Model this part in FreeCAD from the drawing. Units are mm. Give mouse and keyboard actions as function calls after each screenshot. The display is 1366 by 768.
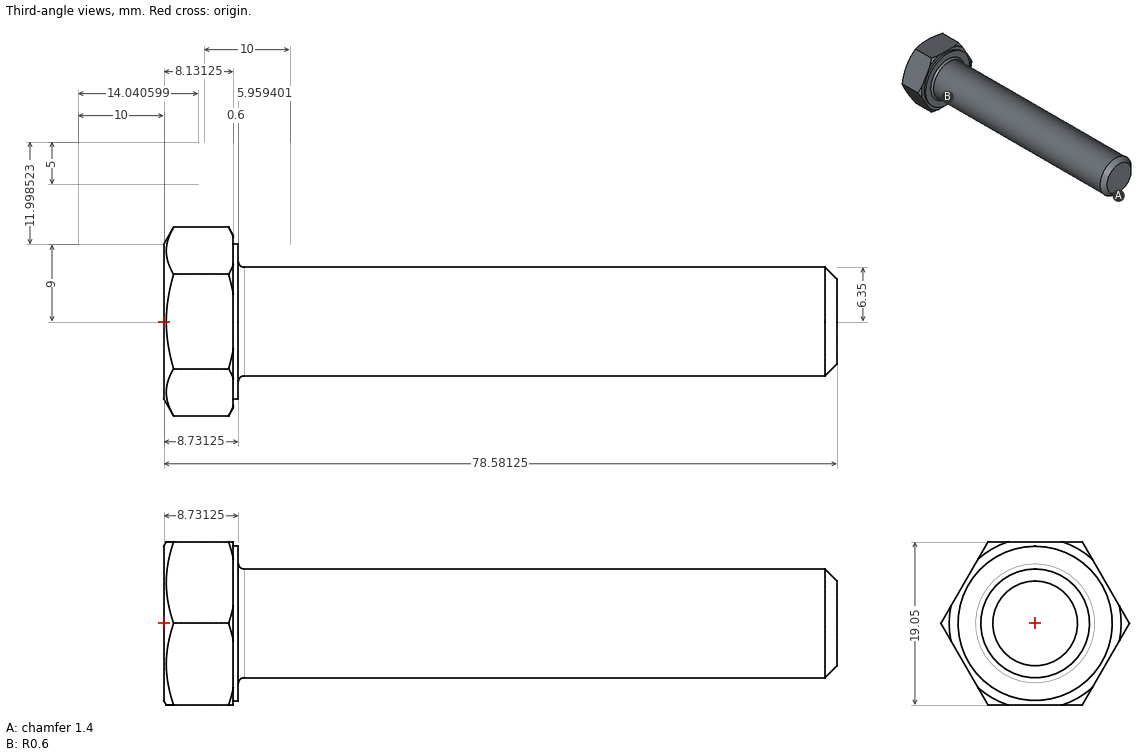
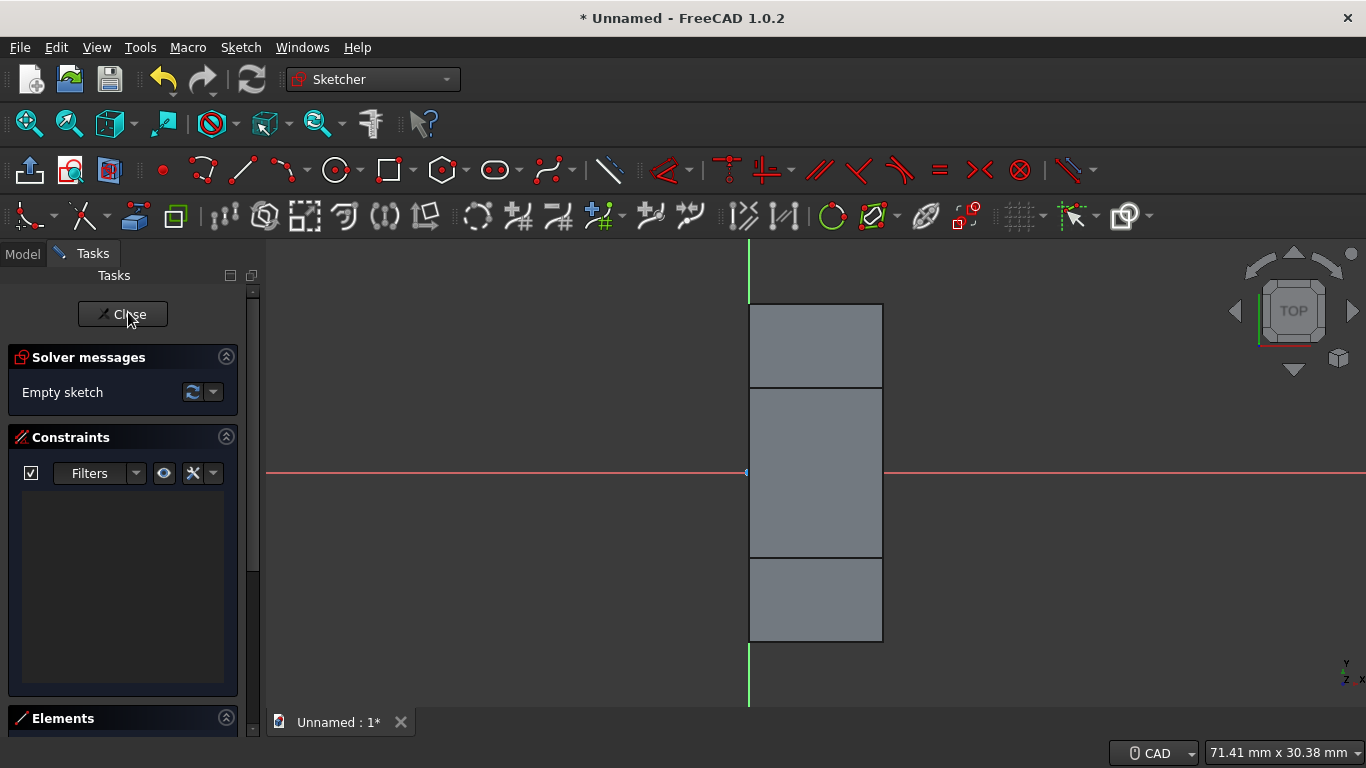
click(110, 170)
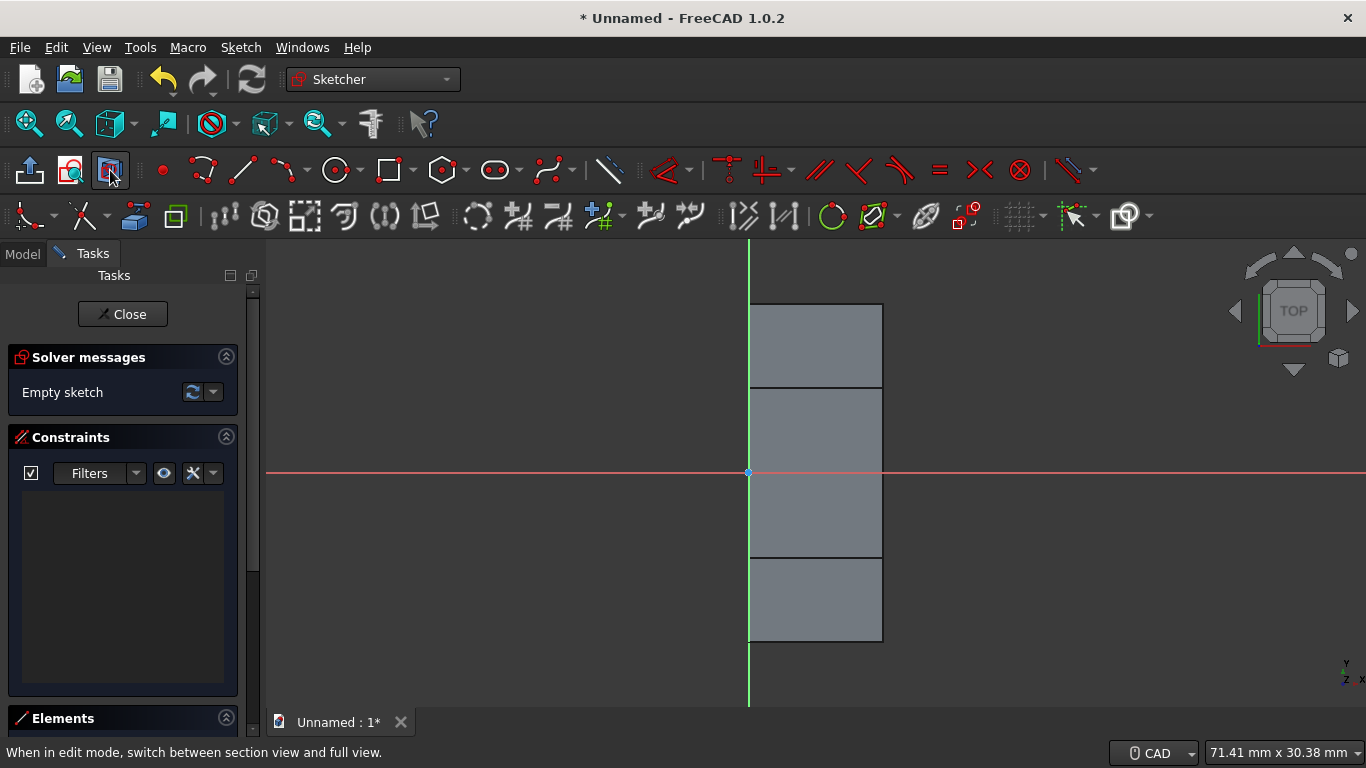
scroll(294, 513, down, 4)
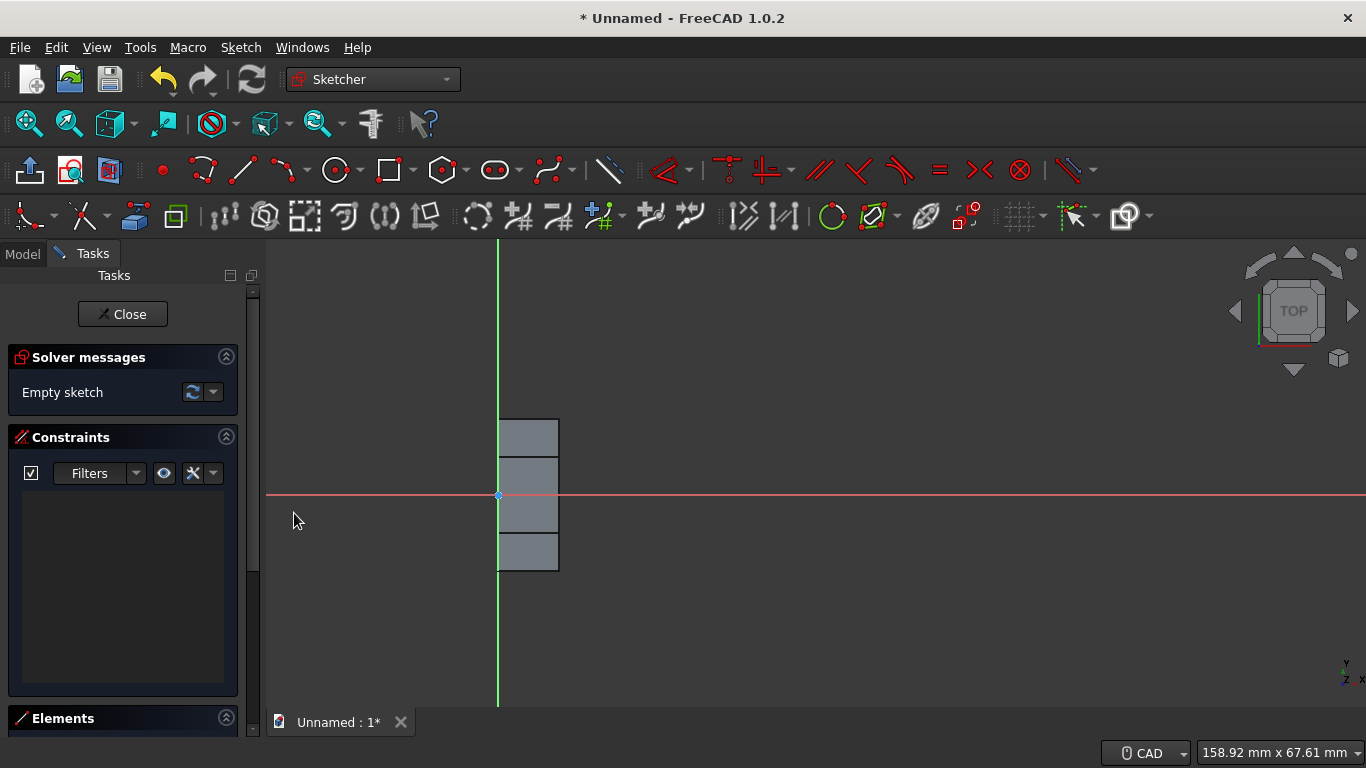
click(390, 170)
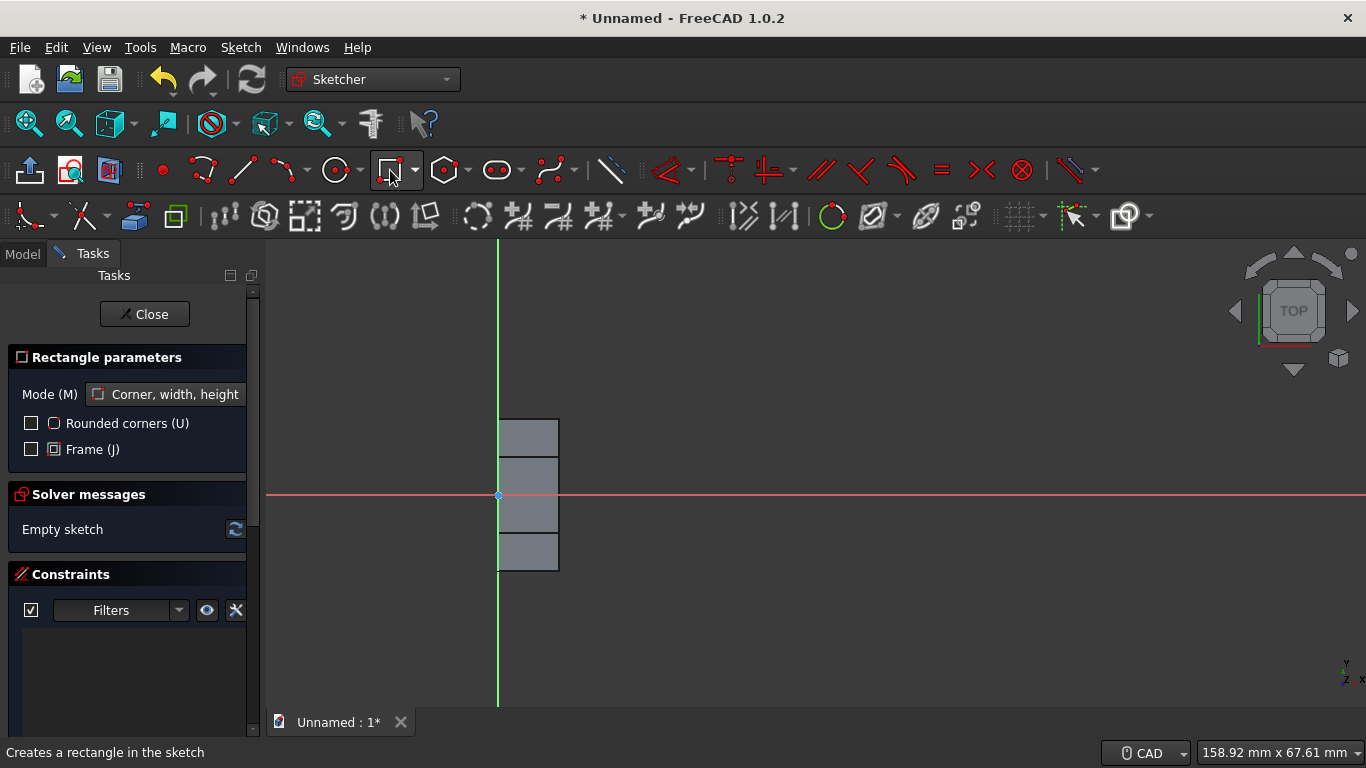
click(498, 495)
move(1042, 451)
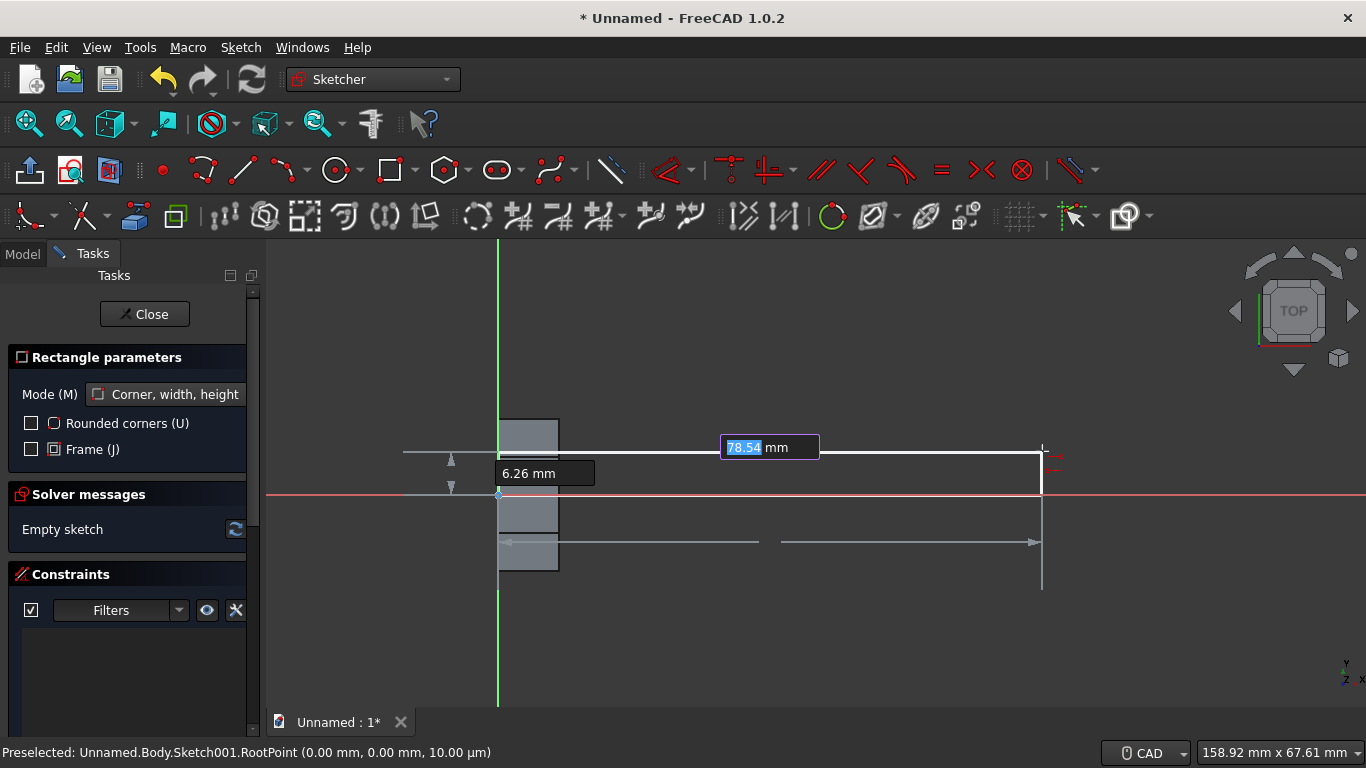
text(78.58125)
key(Tab)
text(6.35)
key(Return)
key(Escape)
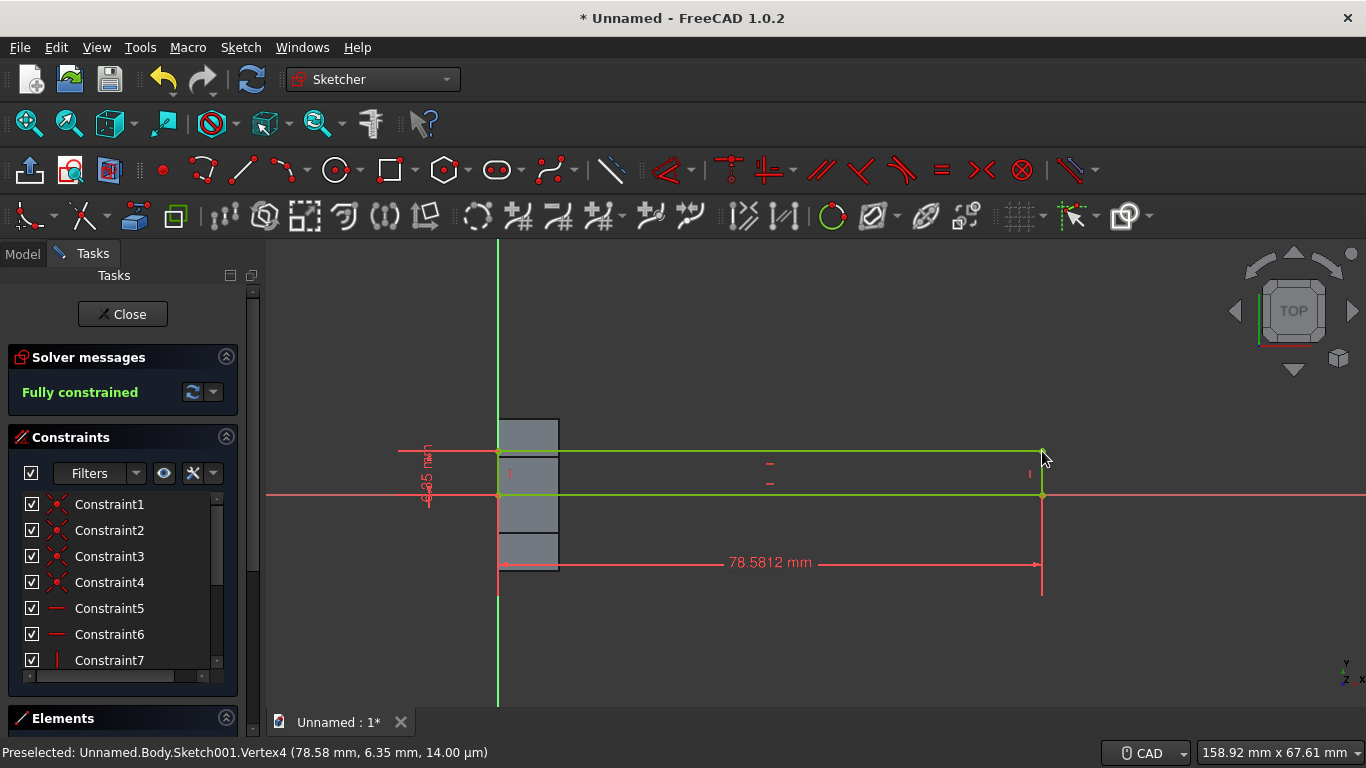
click(123, 314)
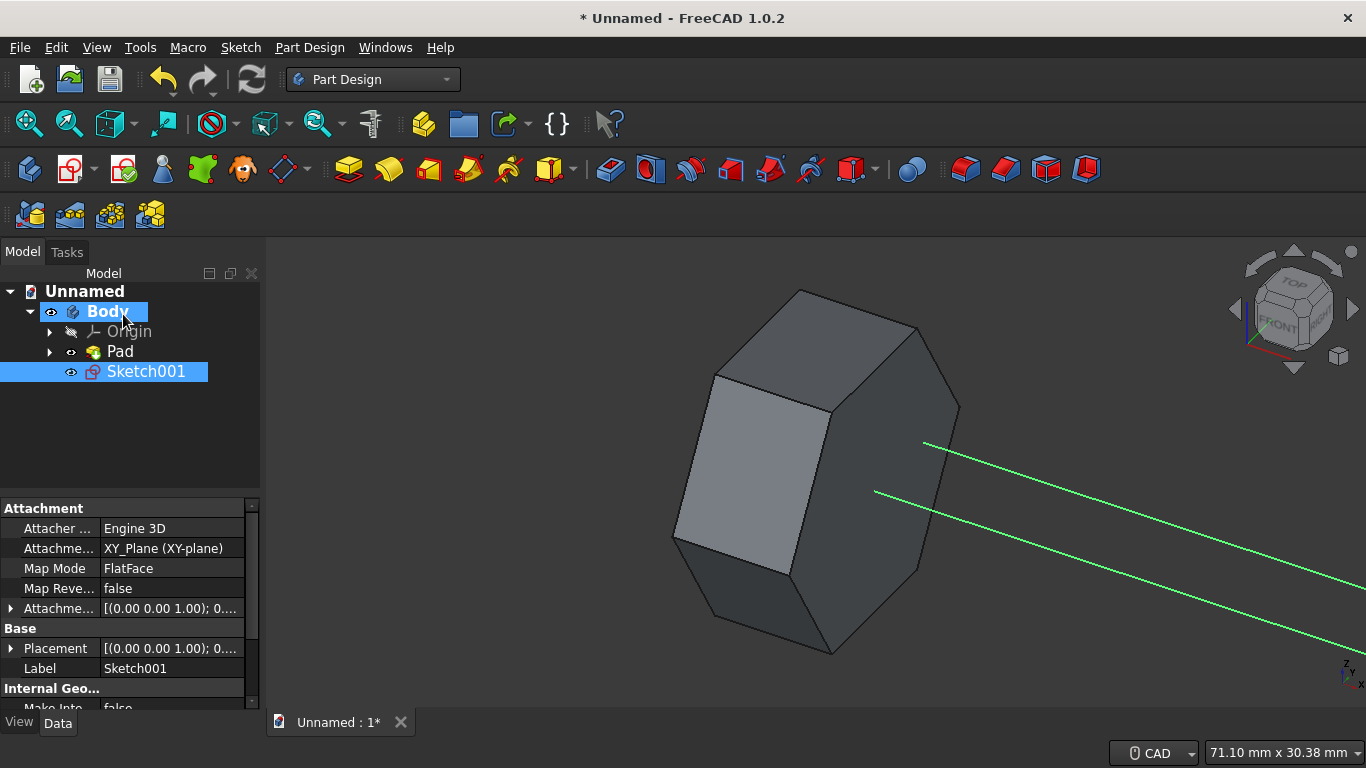
click(390, 170)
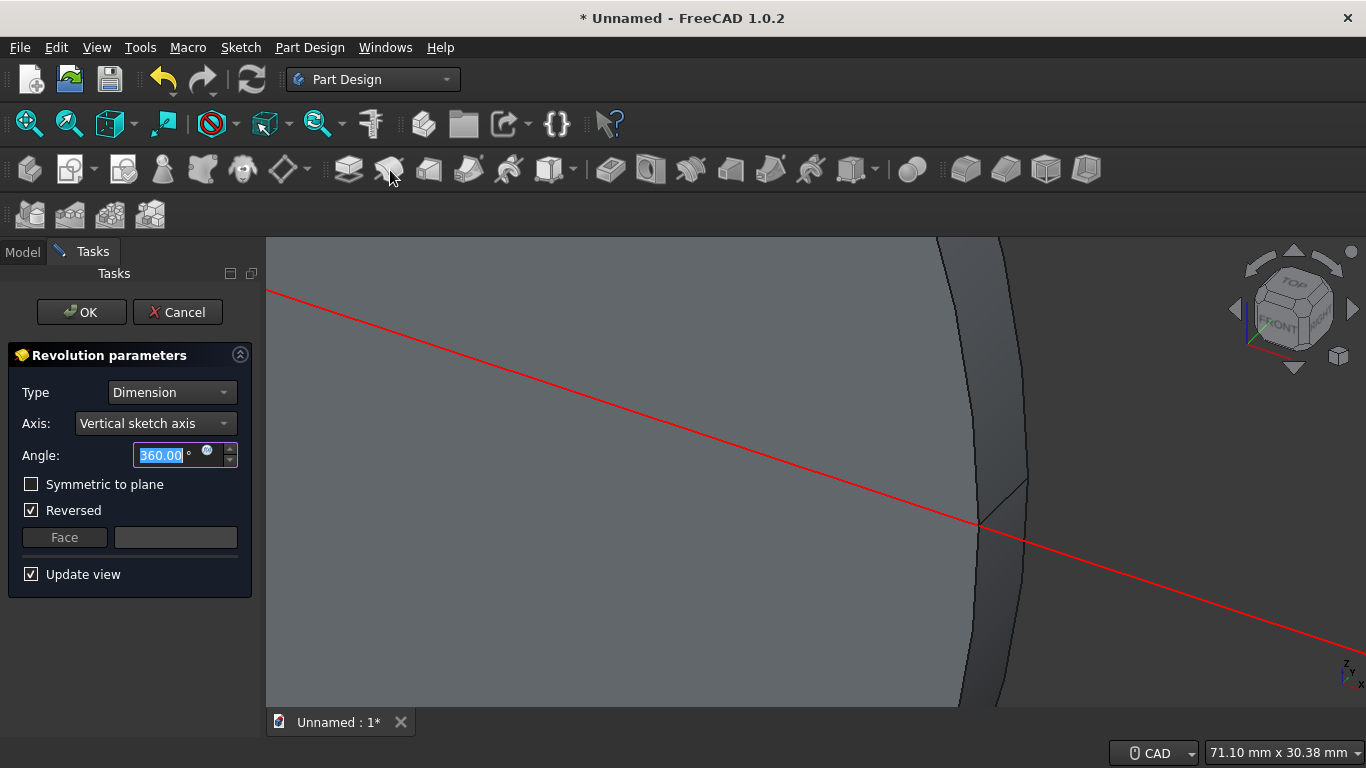
click(156, 424)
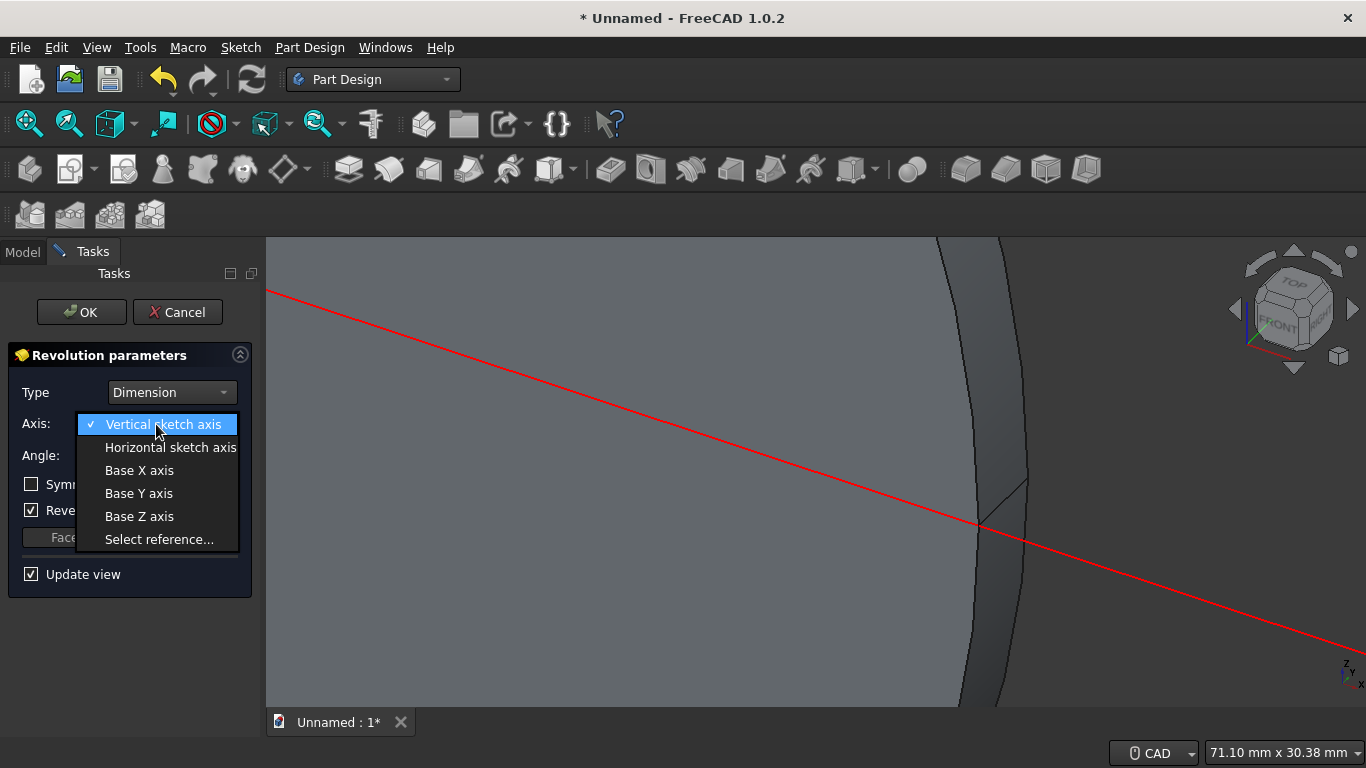
click(156, 448)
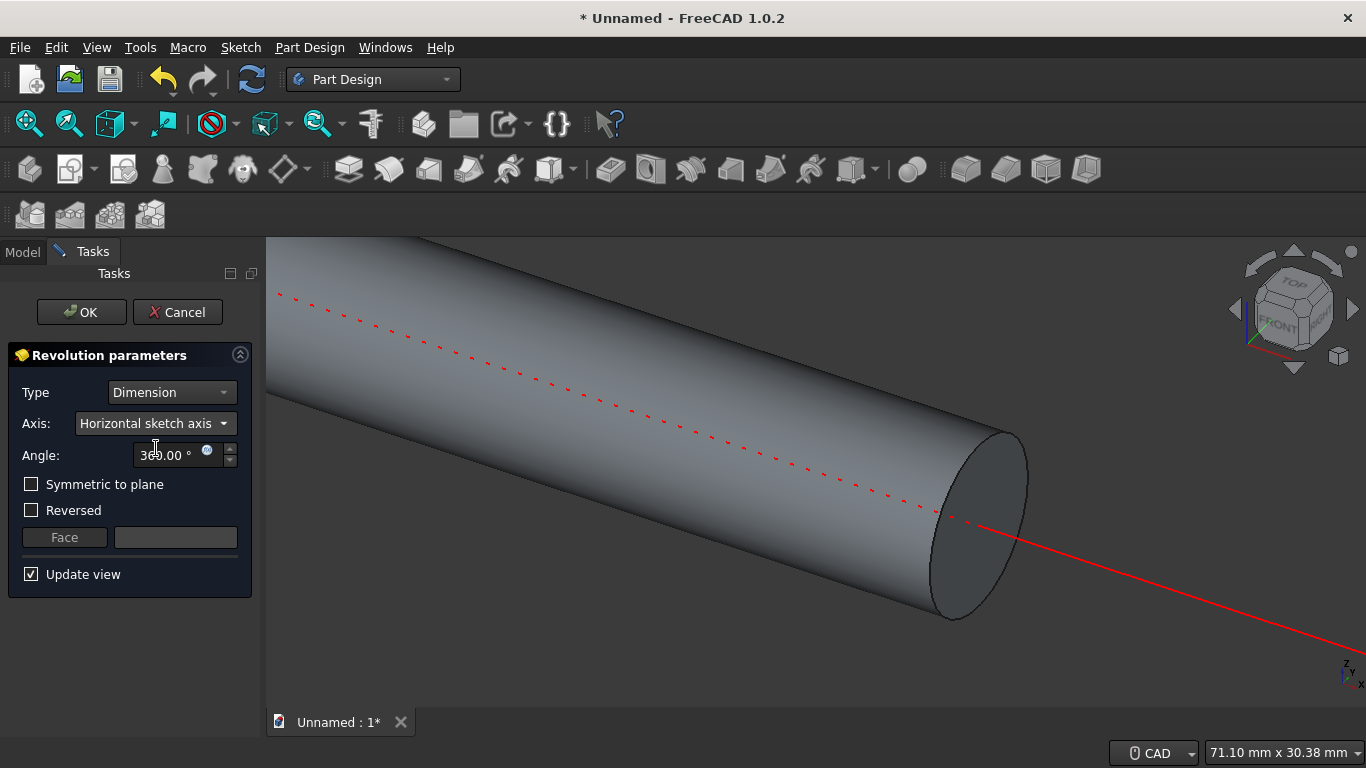
click(82, 312)